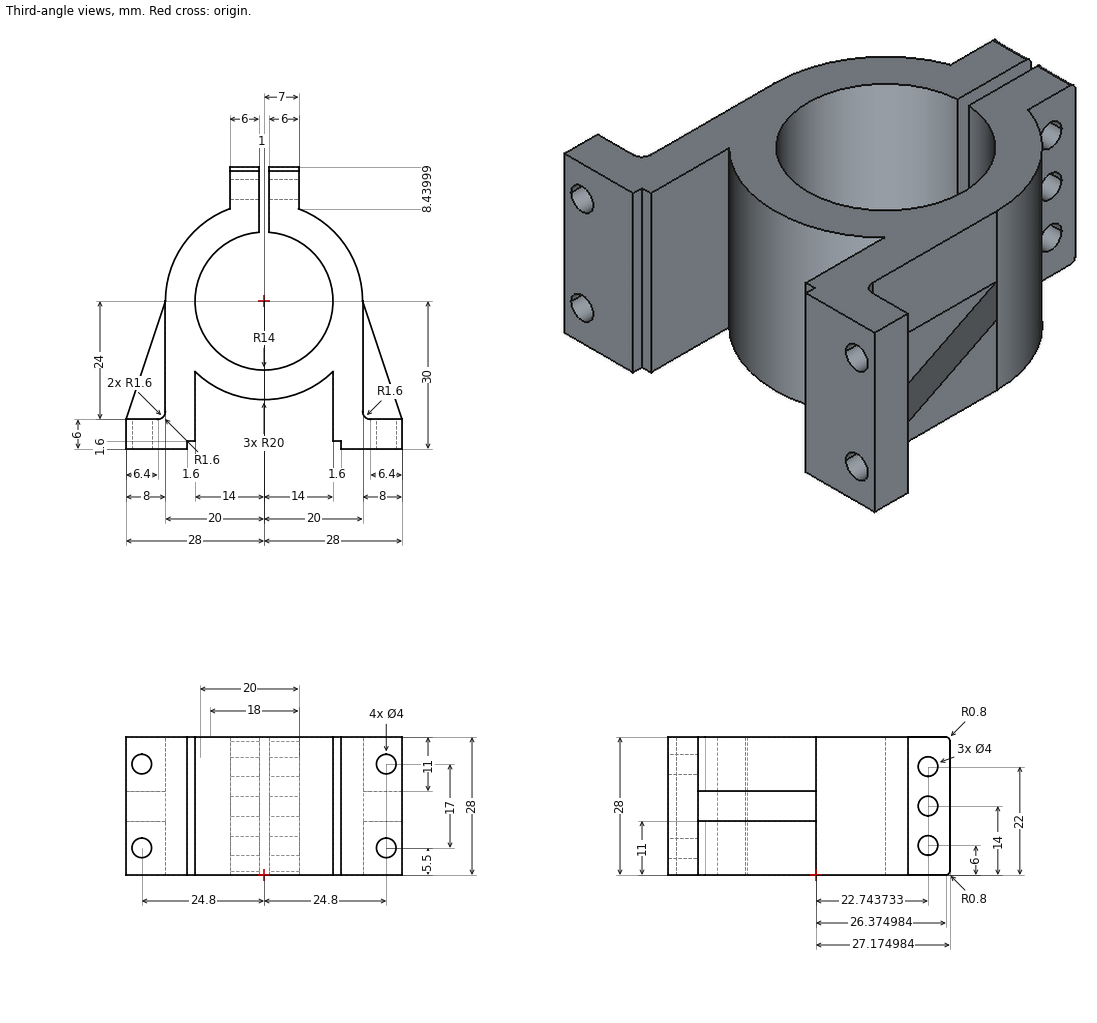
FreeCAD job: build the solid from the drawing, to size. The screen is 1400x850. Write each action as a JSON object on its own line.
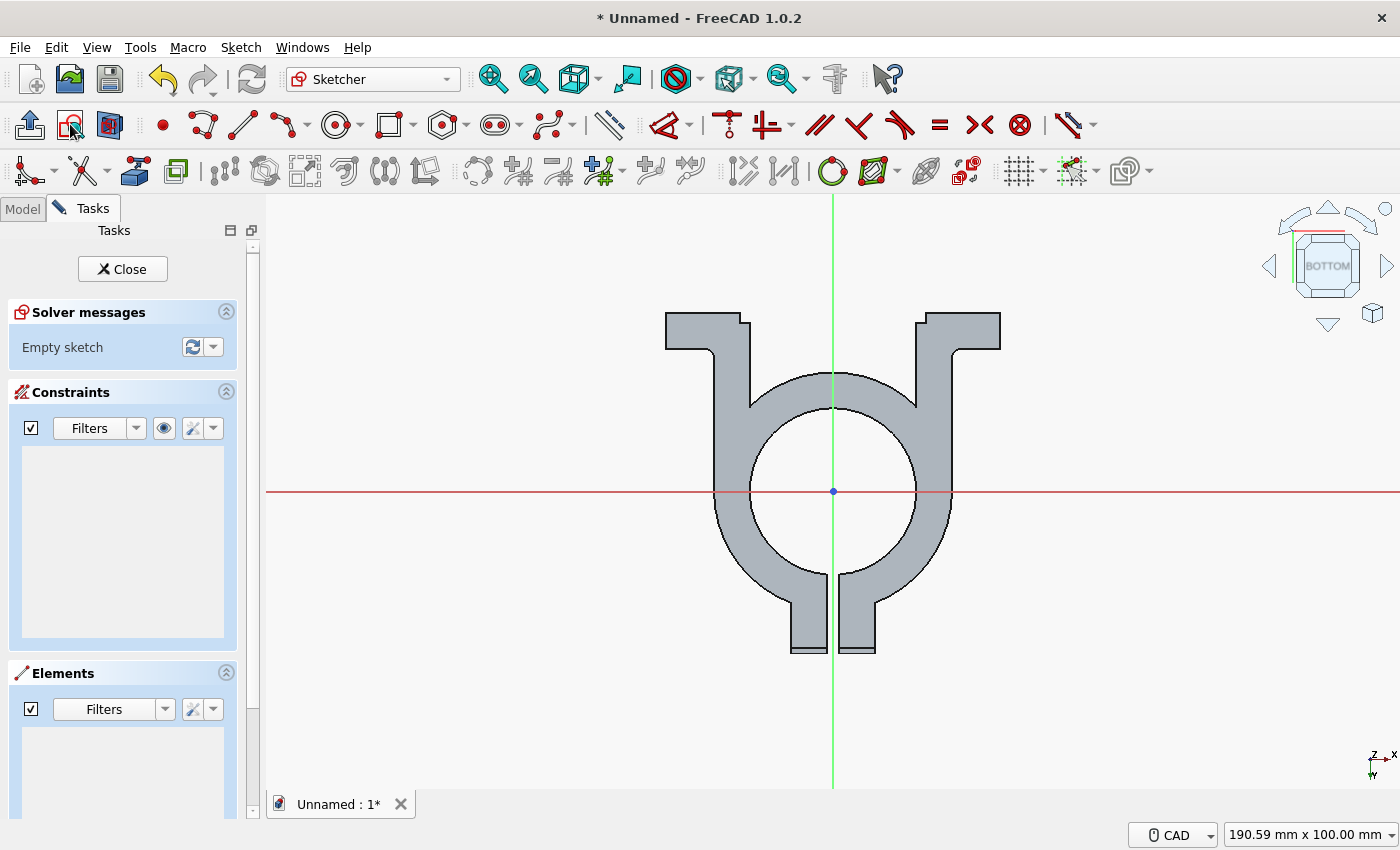
{"action": "scroll", "coordinate": [1005, 379], "scroll_direction": "up", "scroll_amount": 5}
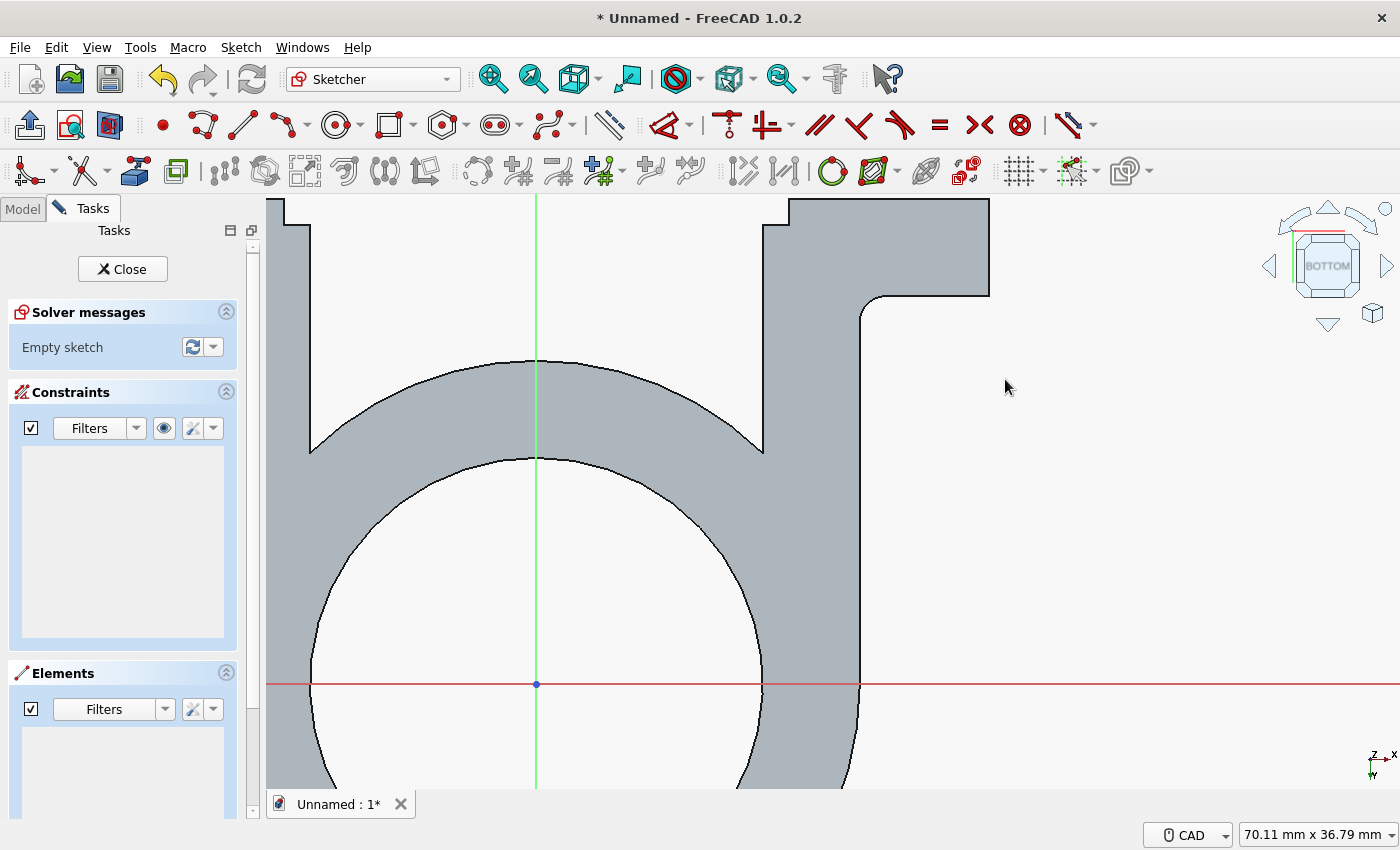
{"action": "left_click", "coordinate": [204, 126]}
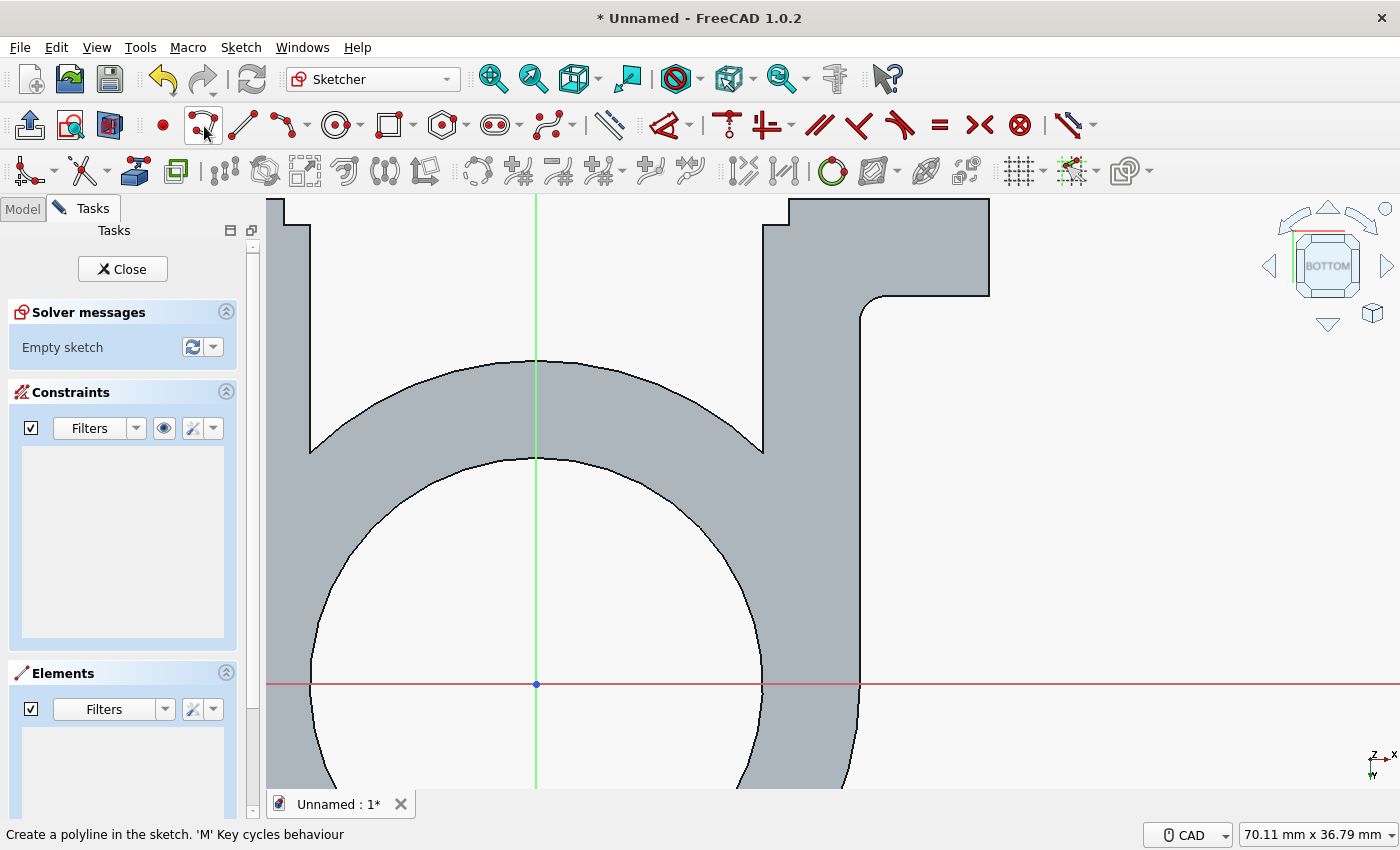
{"action": "left_click", "coordinate": [886, 296]}
{"action": "left_click", "coordinate": [989, 296]}
{"action": "left_click", "coordinate": [860, 684]}
{"action": "left_click", "coordinate": [860, 322]}
{"action": "right_click", "coordinate": [860, 322]}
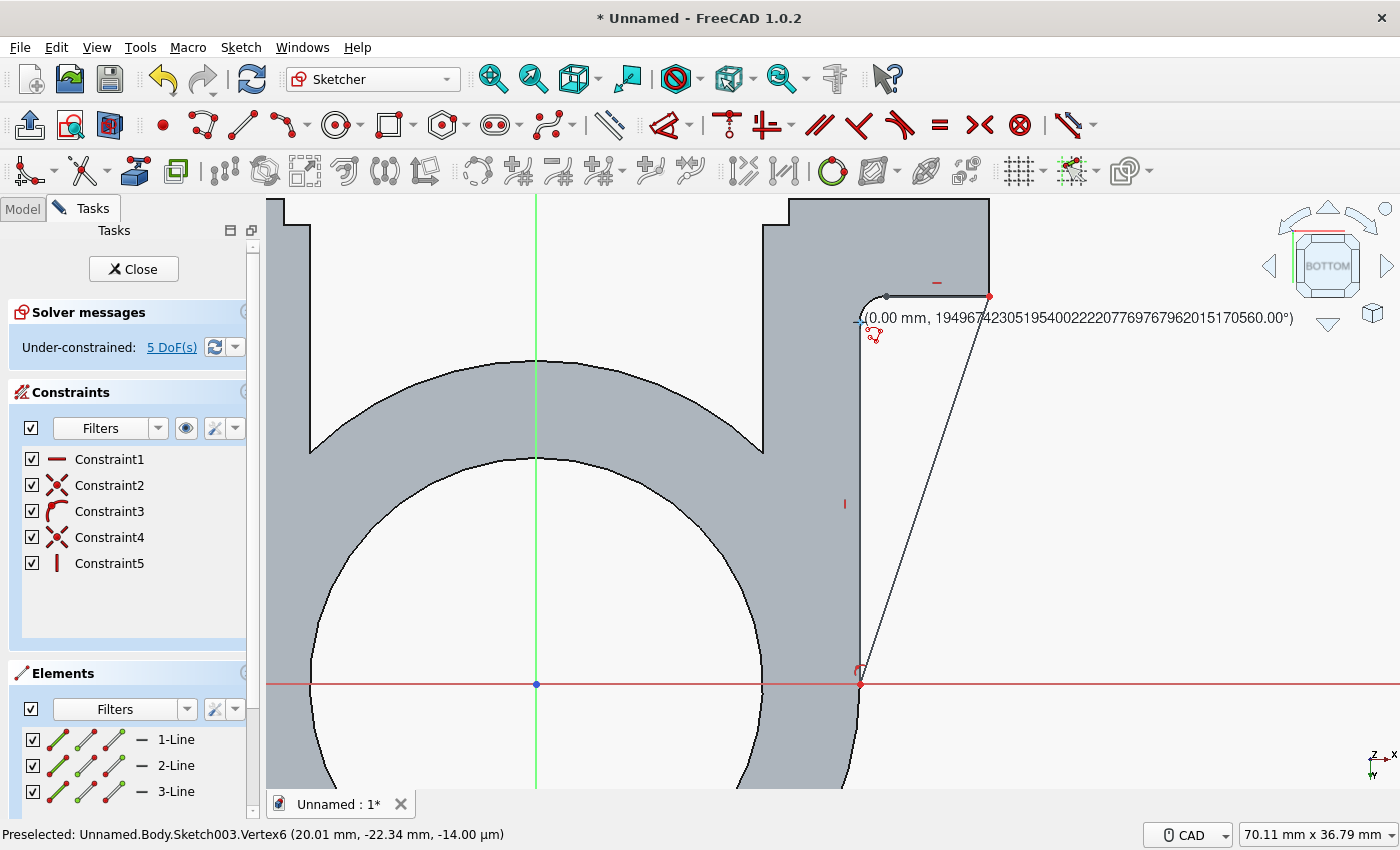
{"action": "left_click", "coordinate": [284, 126]}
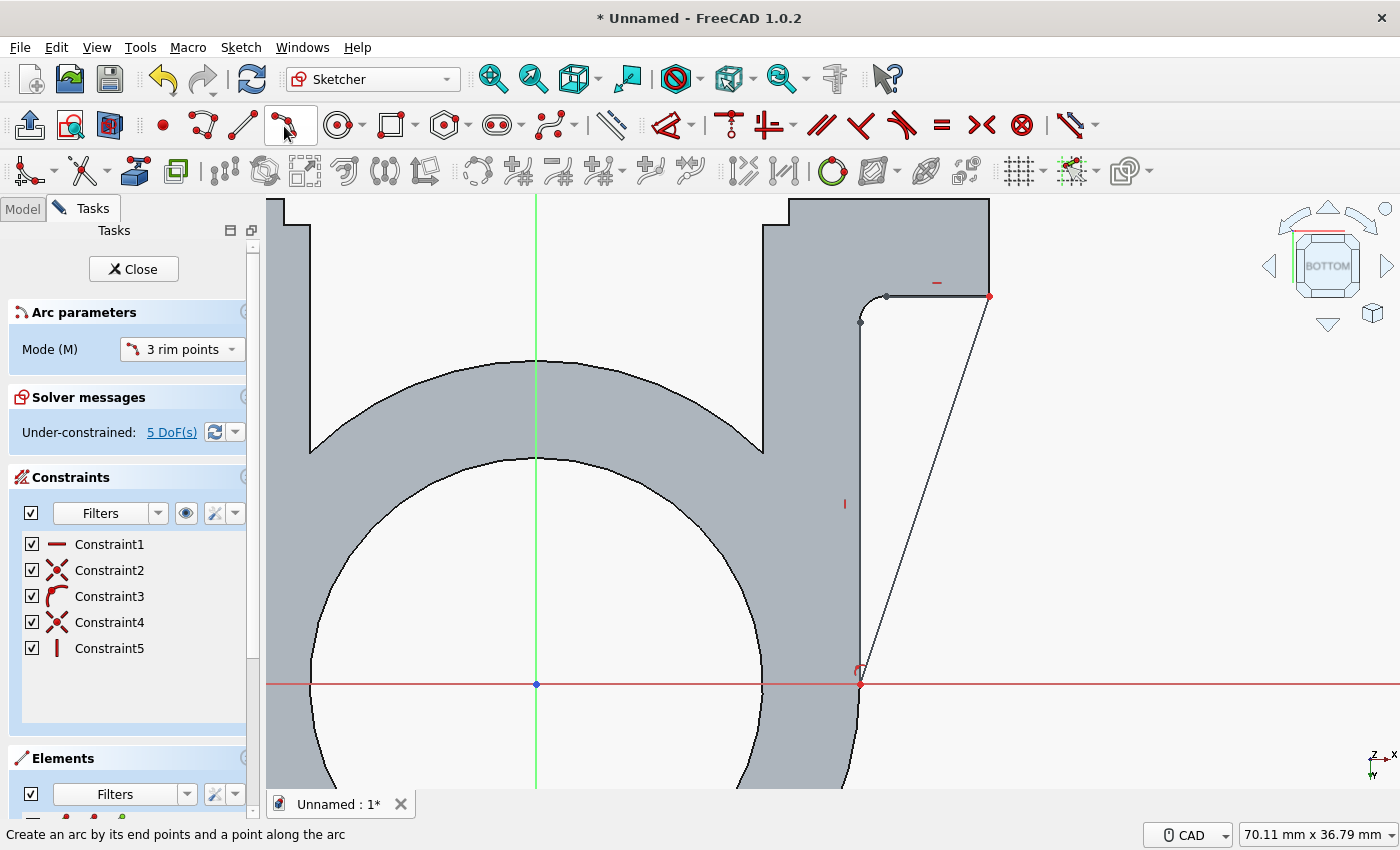
{"action": "left_click", "coordinate": [860, 323]}
{"action": "left_click", "coordinate": [886, 297]}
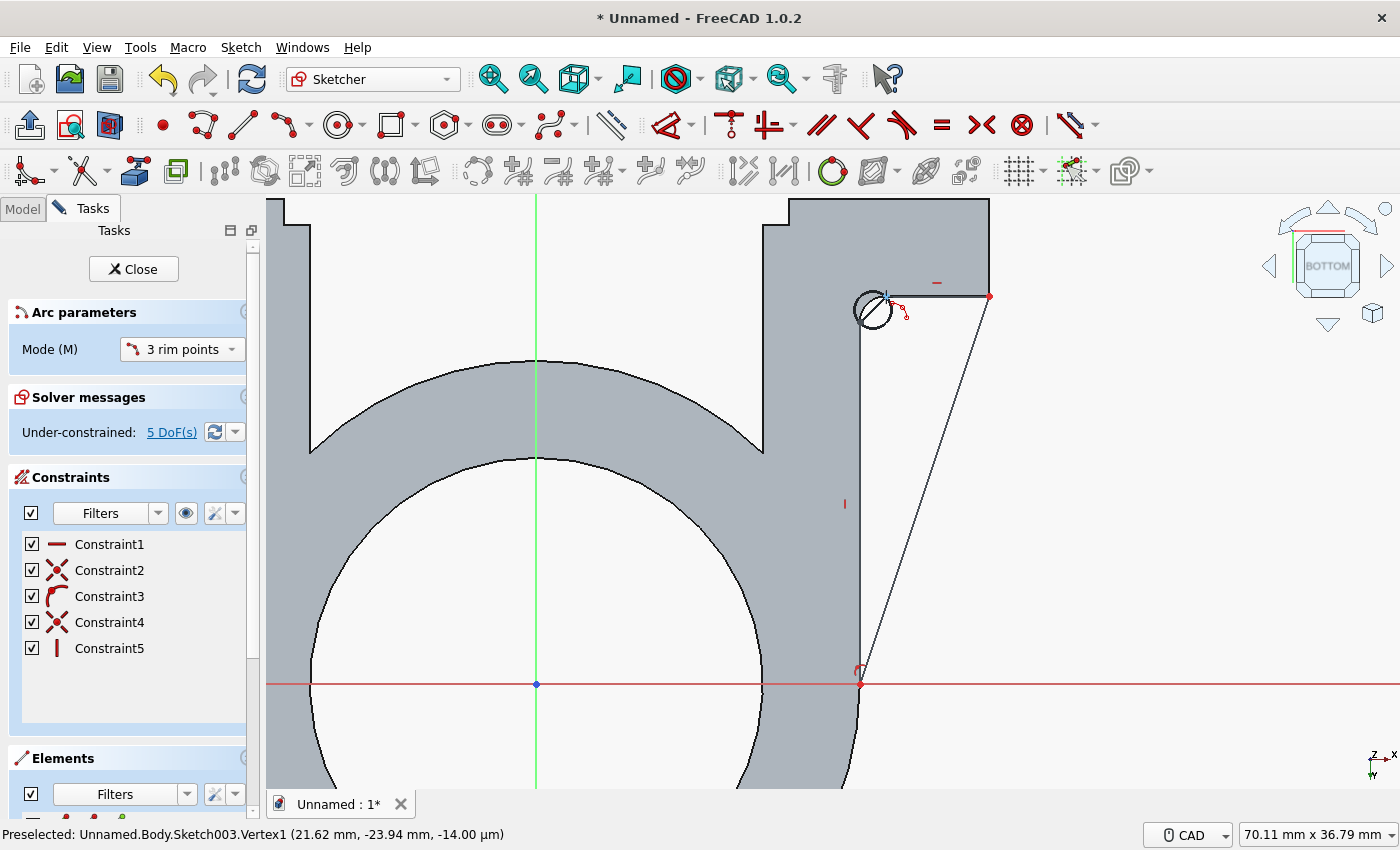
{"action": "scroll", "coordinate": [867, 304], "scroll_direction": "up", "scroll_amount": 4}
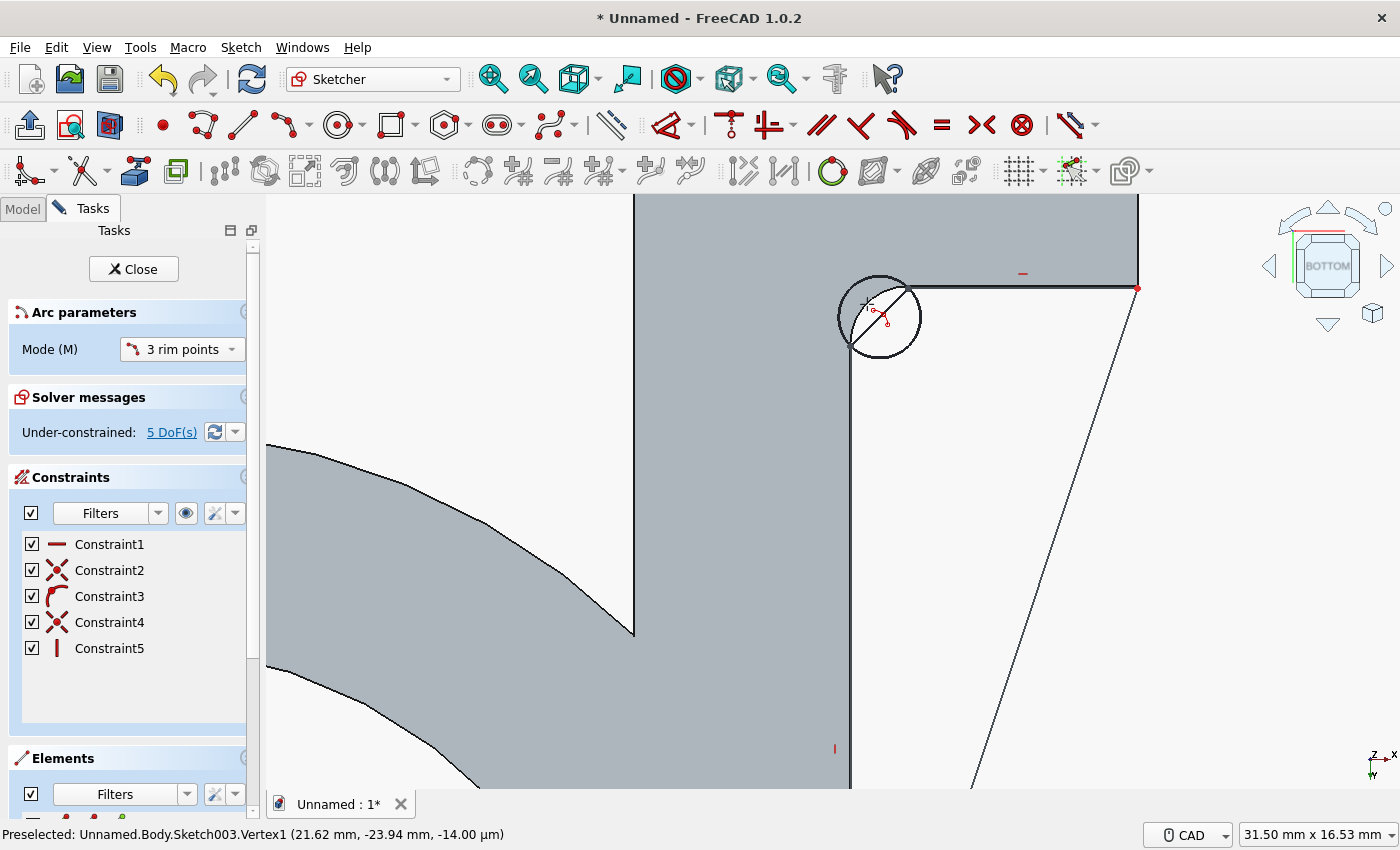
{"action": "left_click", "coordinate": [867, 303]}
{"action": "key", "text": "Escape"}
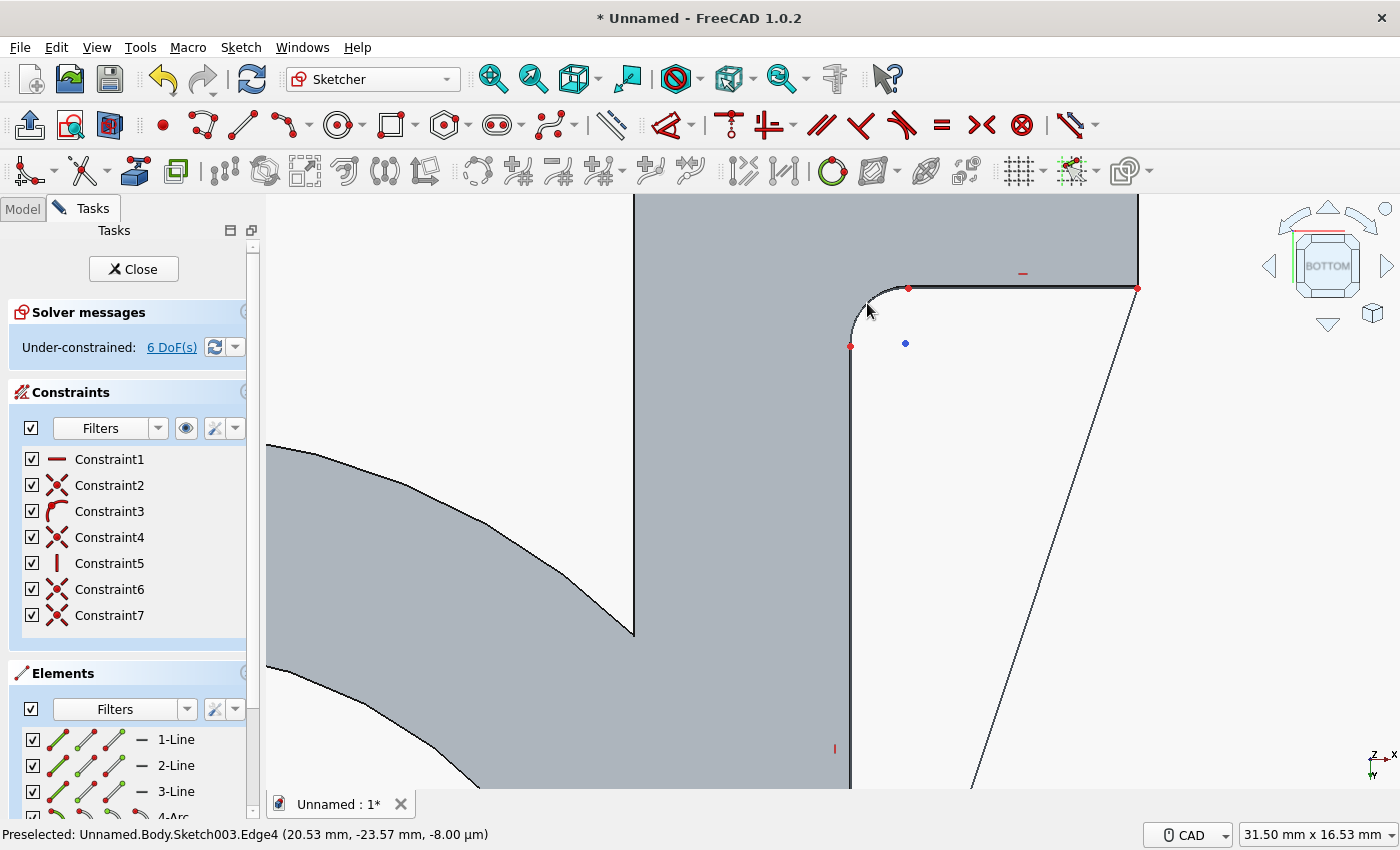
{"action": "left_click", "coordinate": [977, 288]}